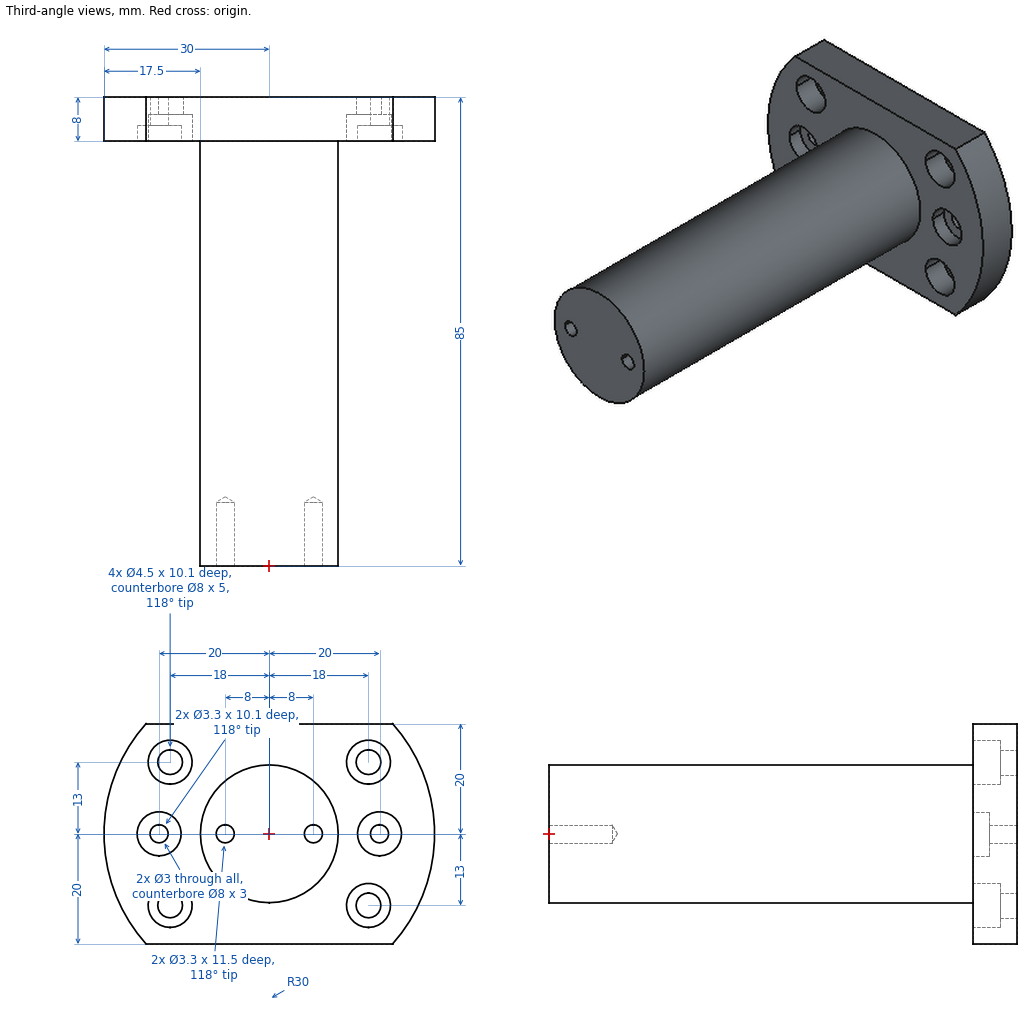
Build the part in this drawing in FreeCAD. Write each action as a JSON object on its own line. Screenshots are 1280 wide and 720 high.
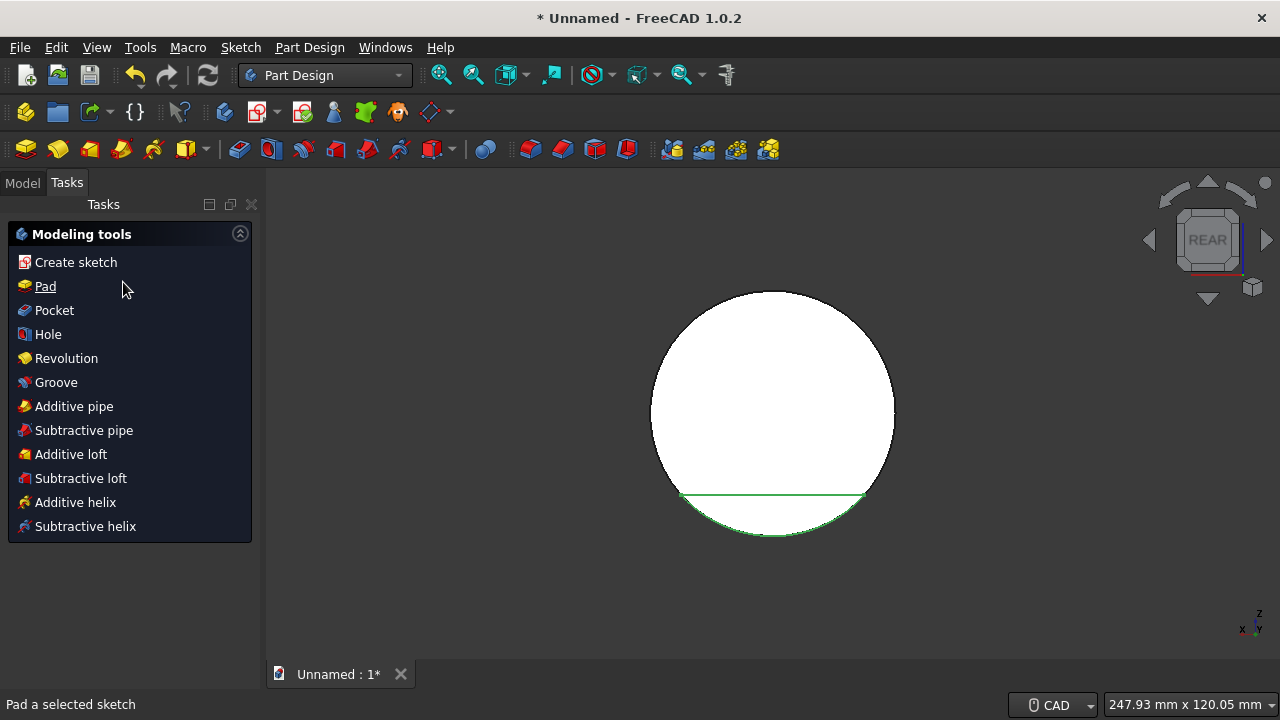
{"action": "left_click", "coordinate": [240, 150]}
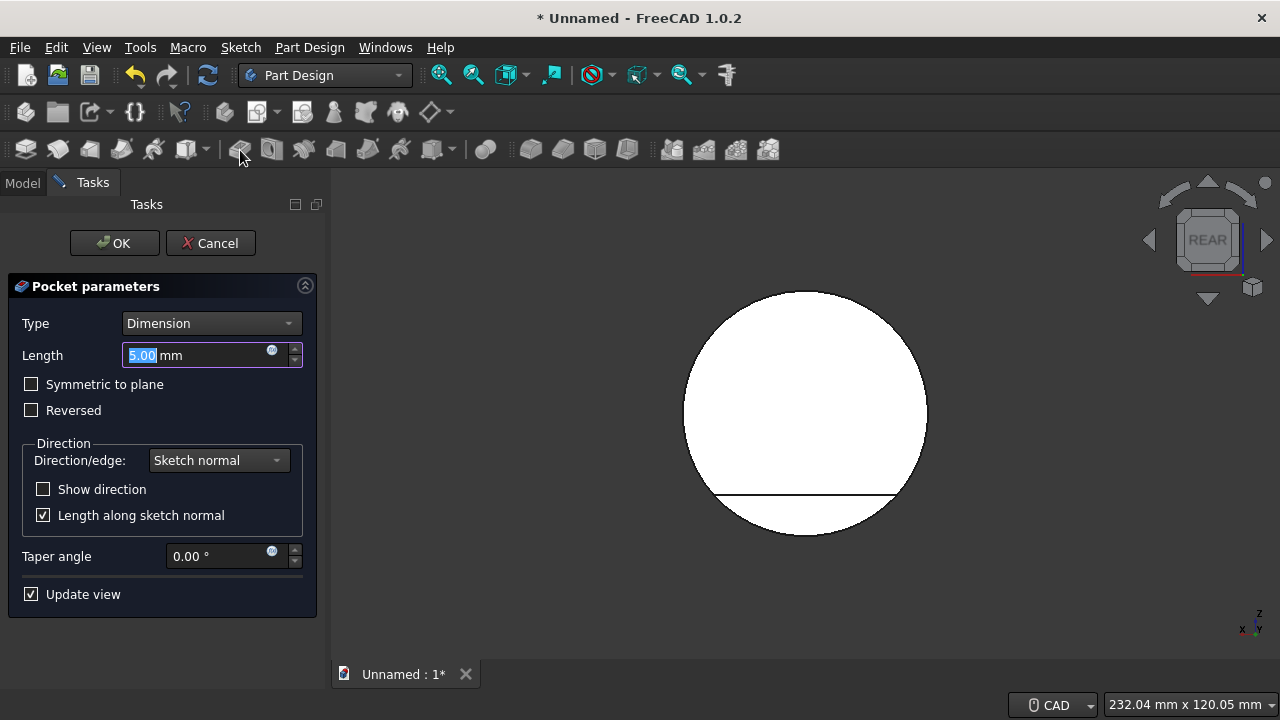
{"action": "left_click", "coordinate": [212, 324]}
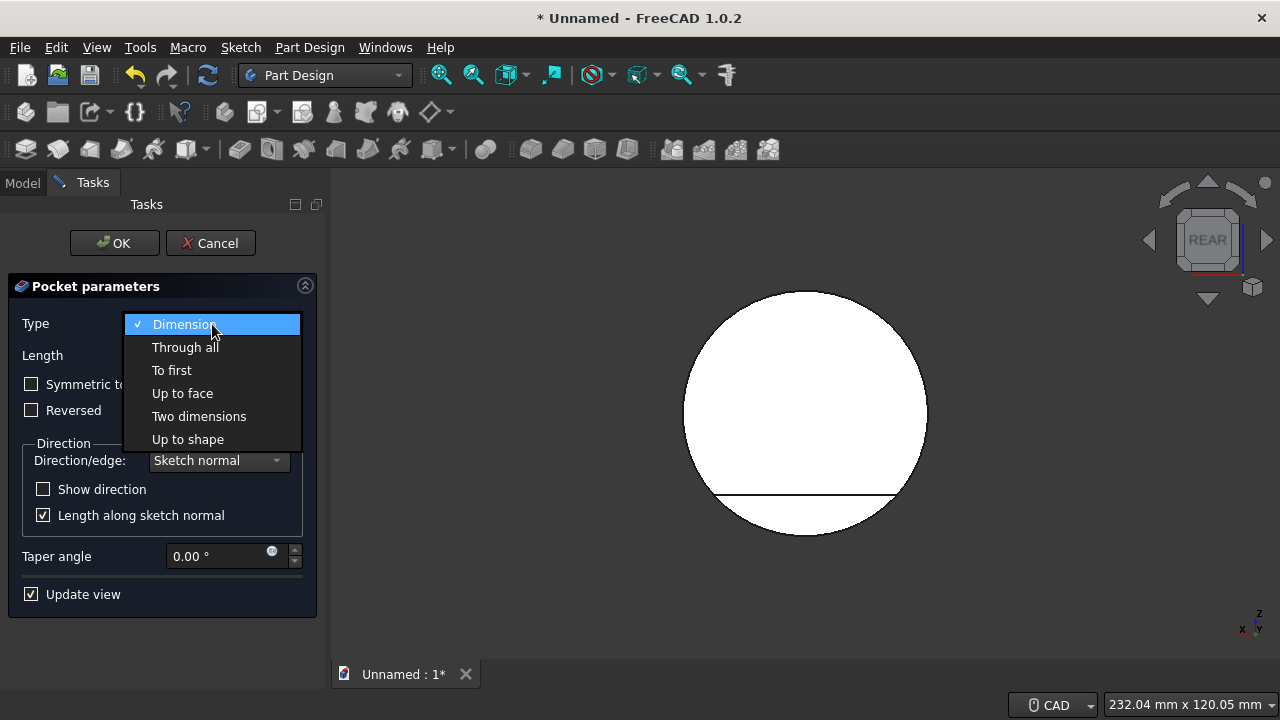
{"action": "left_click", "coordinate": [212, 370]}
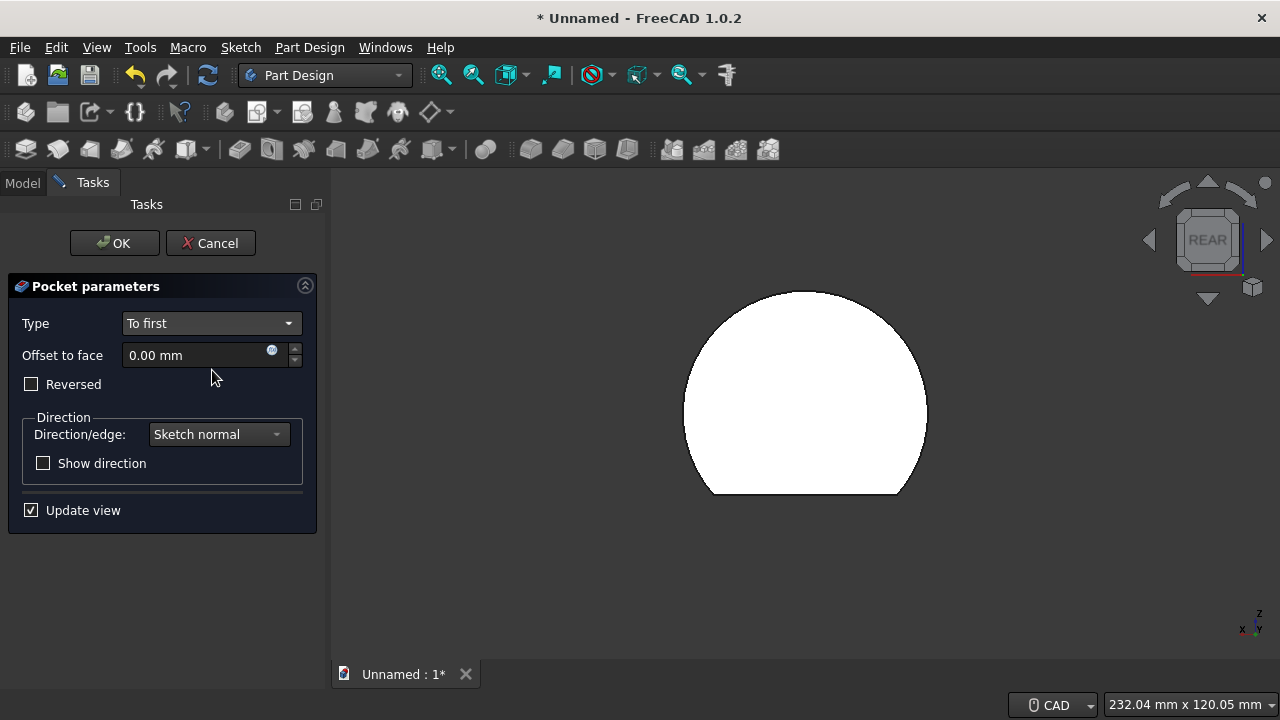
{"action": "left_click", "coordinate": [115, 243]}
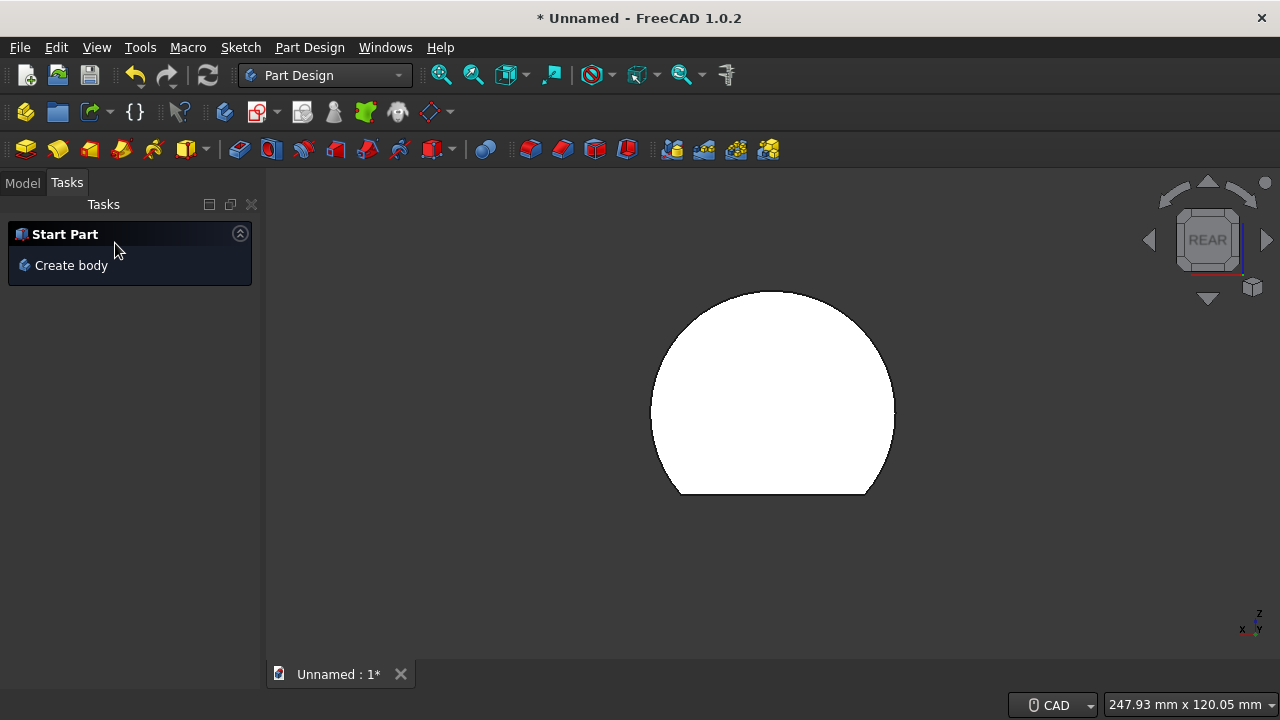
{"action": "left_click", "coordinate": [442, 76]}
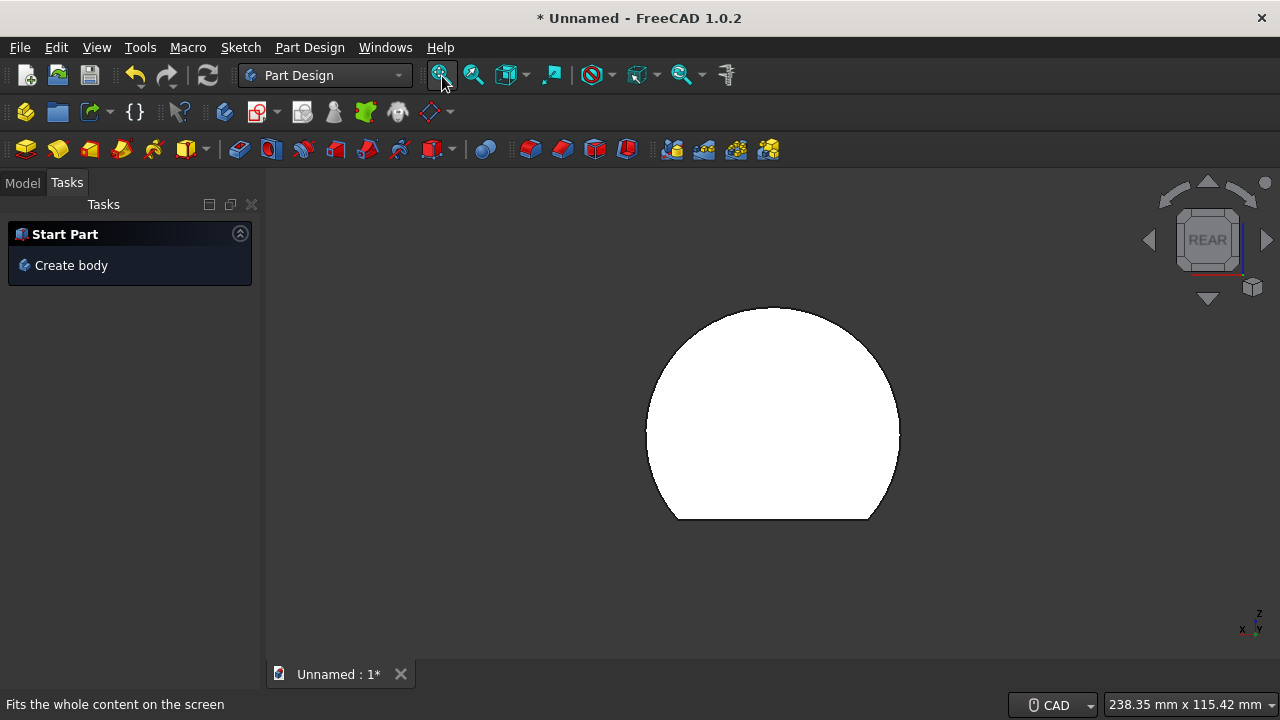
{"action": "left_click", "coordinate": [773, 412]}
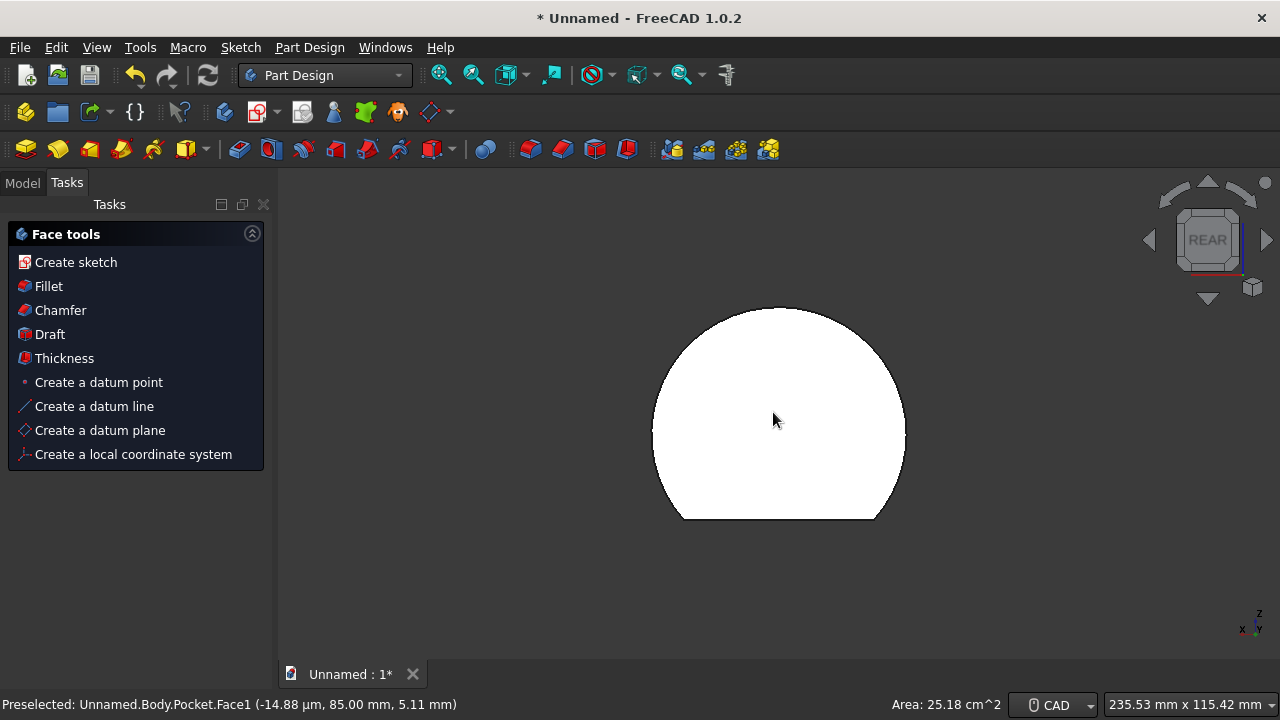
{"action": "left_click", "coordinate": [258, 112]}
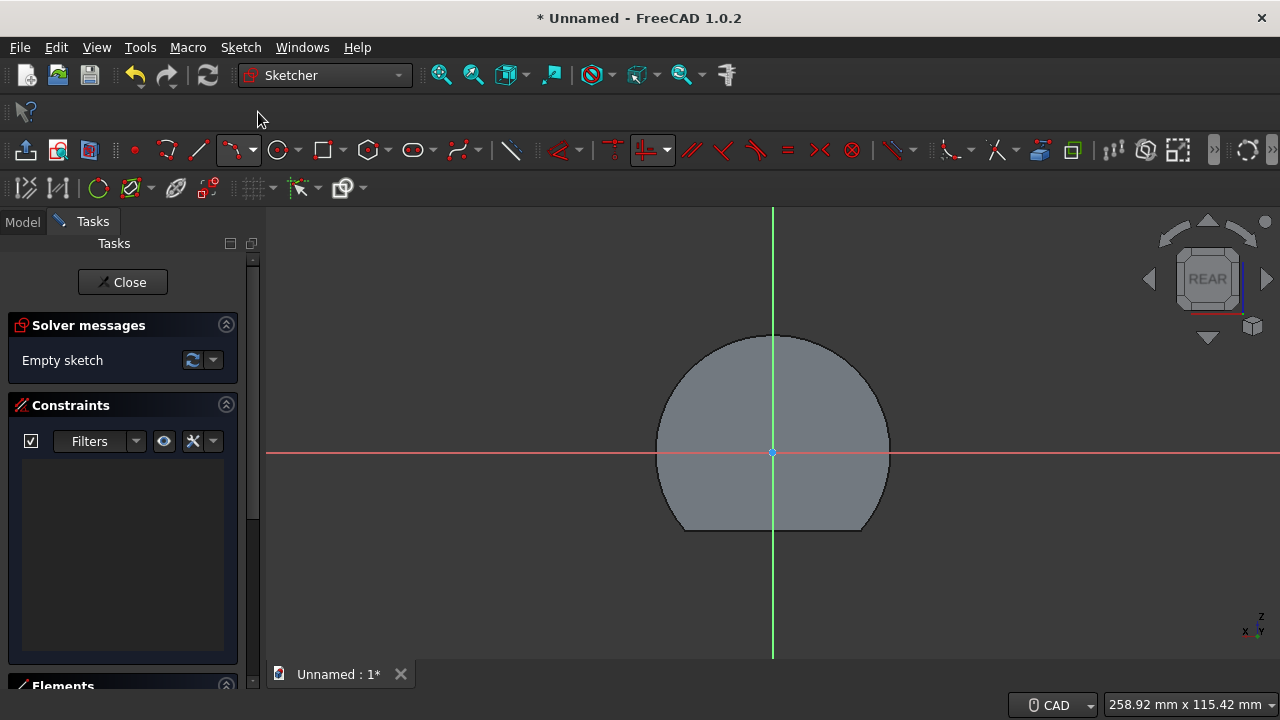
{"action": "scroll", "coordinate": [829, 362], "scroll_direction": "up", "scroll_amount": 4}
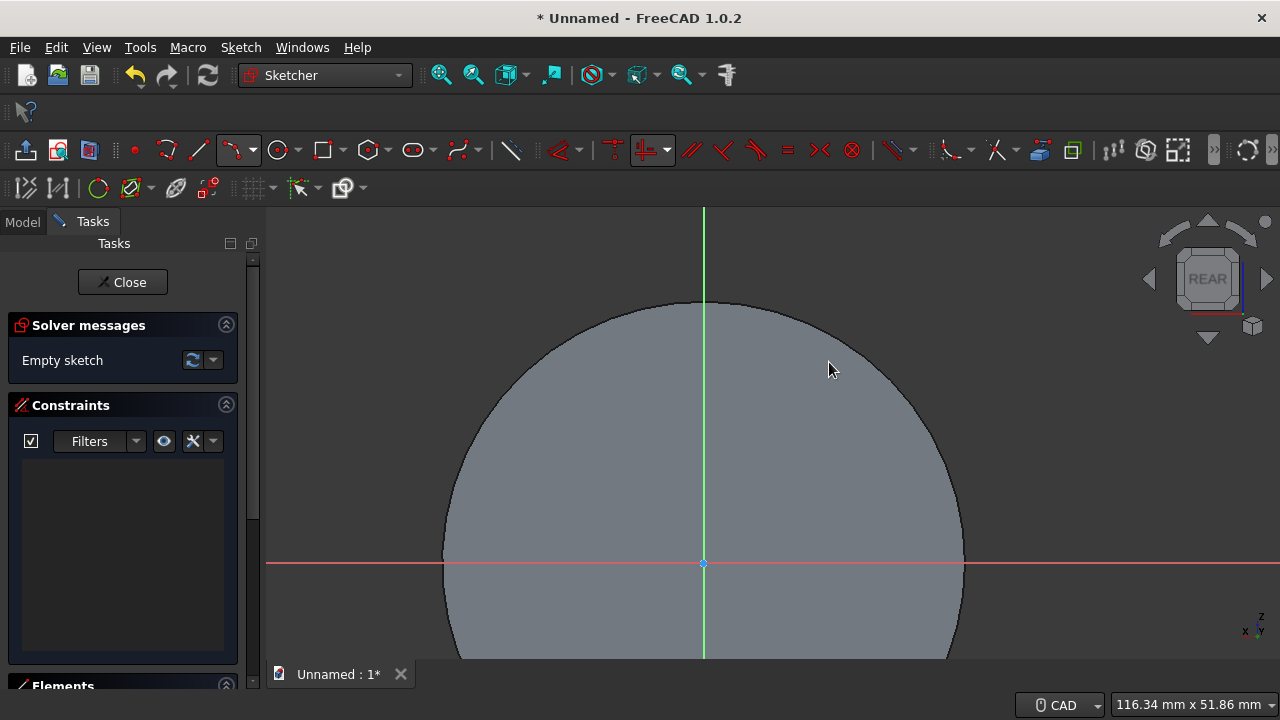
{"action": "left_click", "coordinate": [200, 150]}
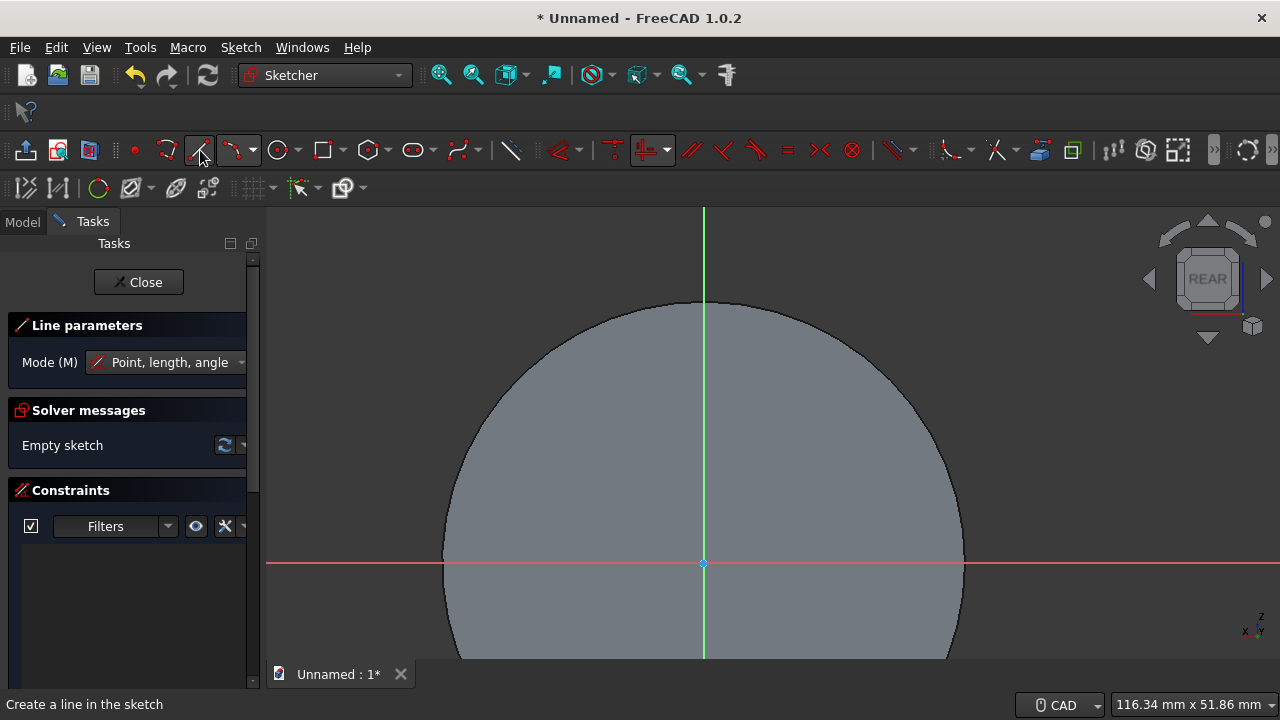
{"action": "left_click", "coordinate": [509, 389]}
{"action": "left_click", "coordinate": [898, 389]}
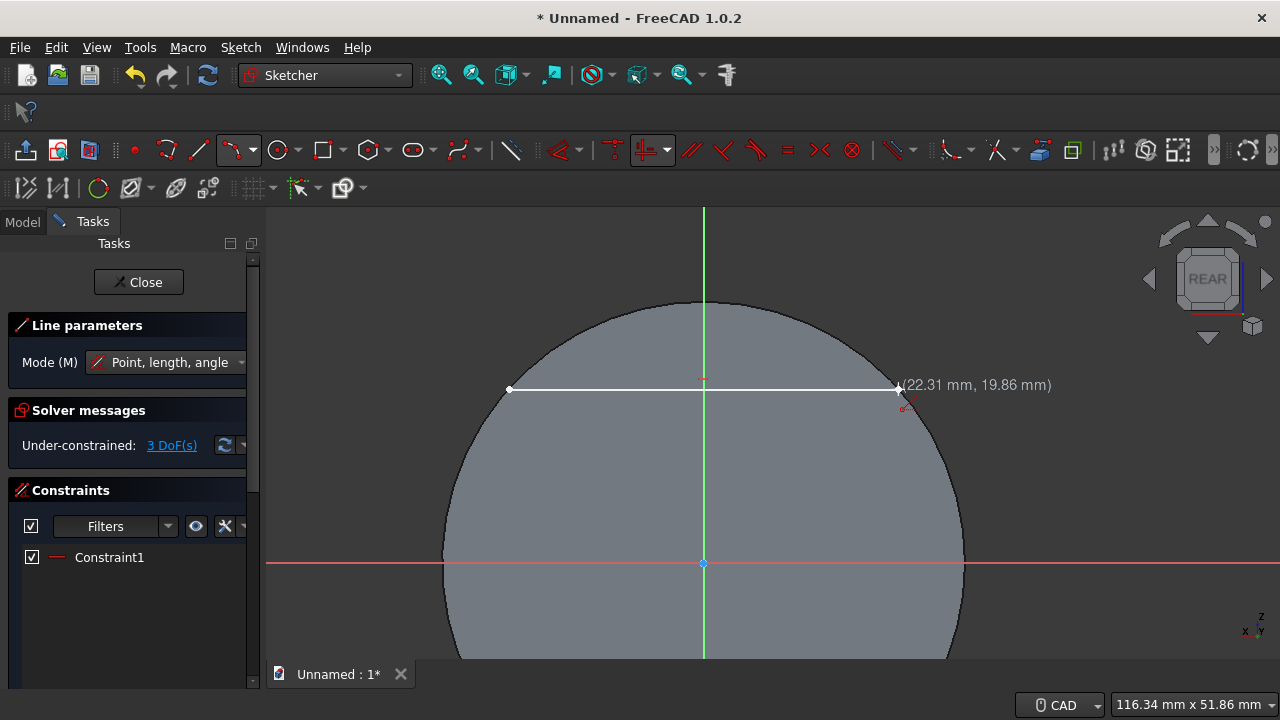
{"action": "left_click", "coordinate": [232, 150]}